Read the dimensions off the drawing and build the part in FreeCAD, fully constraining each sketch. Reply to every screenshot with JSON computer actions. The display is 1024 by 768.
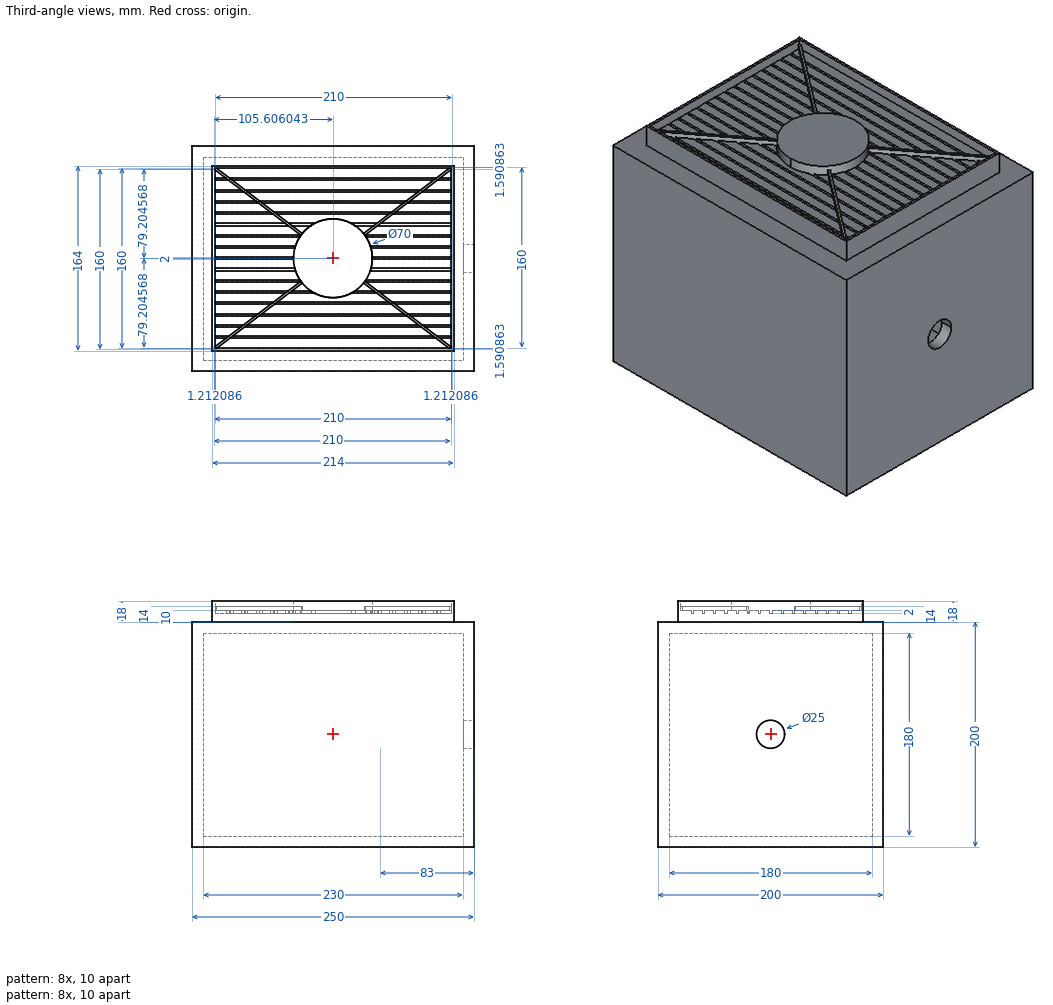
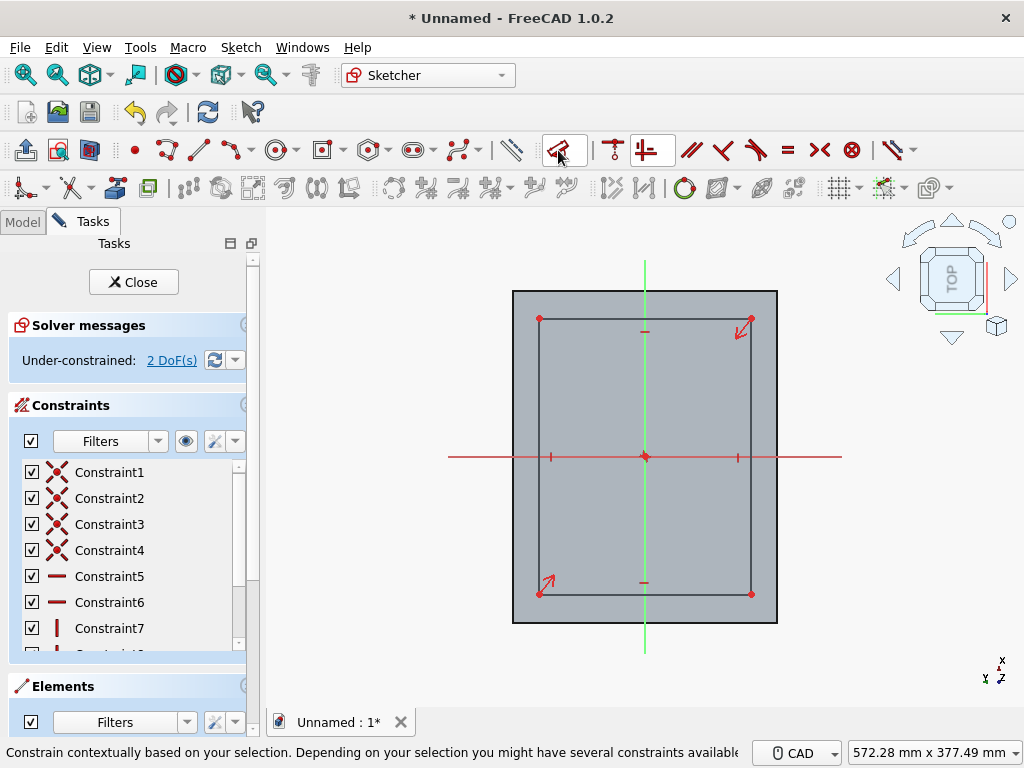
{"action": "left_click", "coordinate": [603, 595]}
{"action": "left_click", "coordinate": [596, 629]}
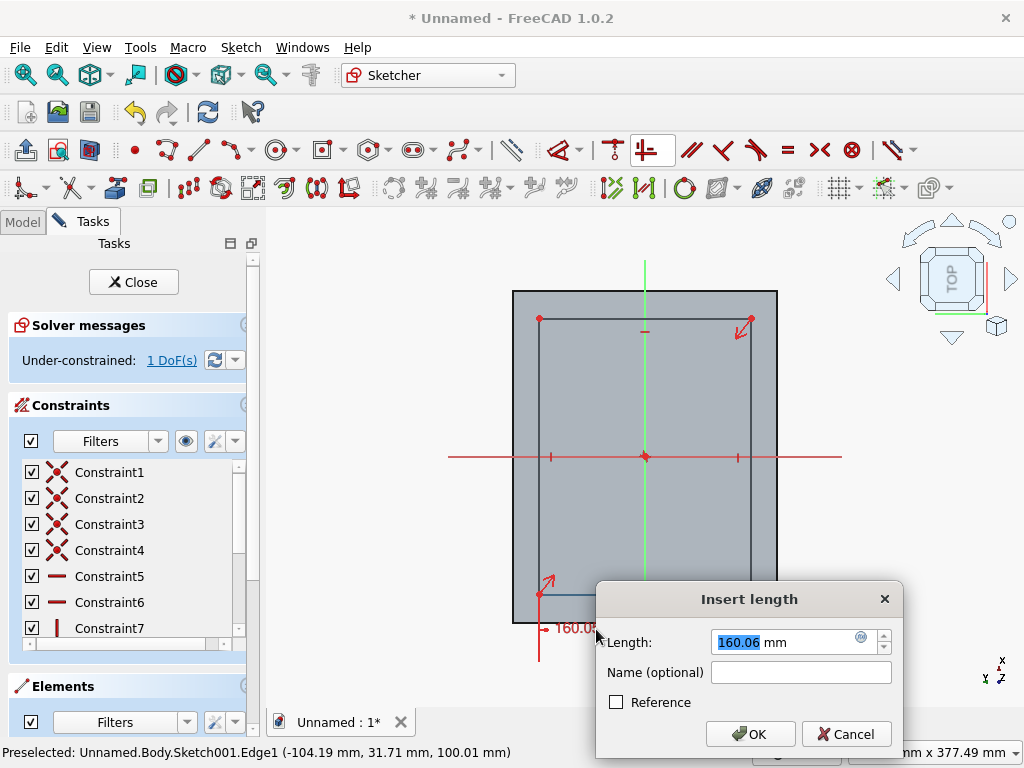
{"action": "type", "text": "160"}
{"action": "key", "text": "Return"}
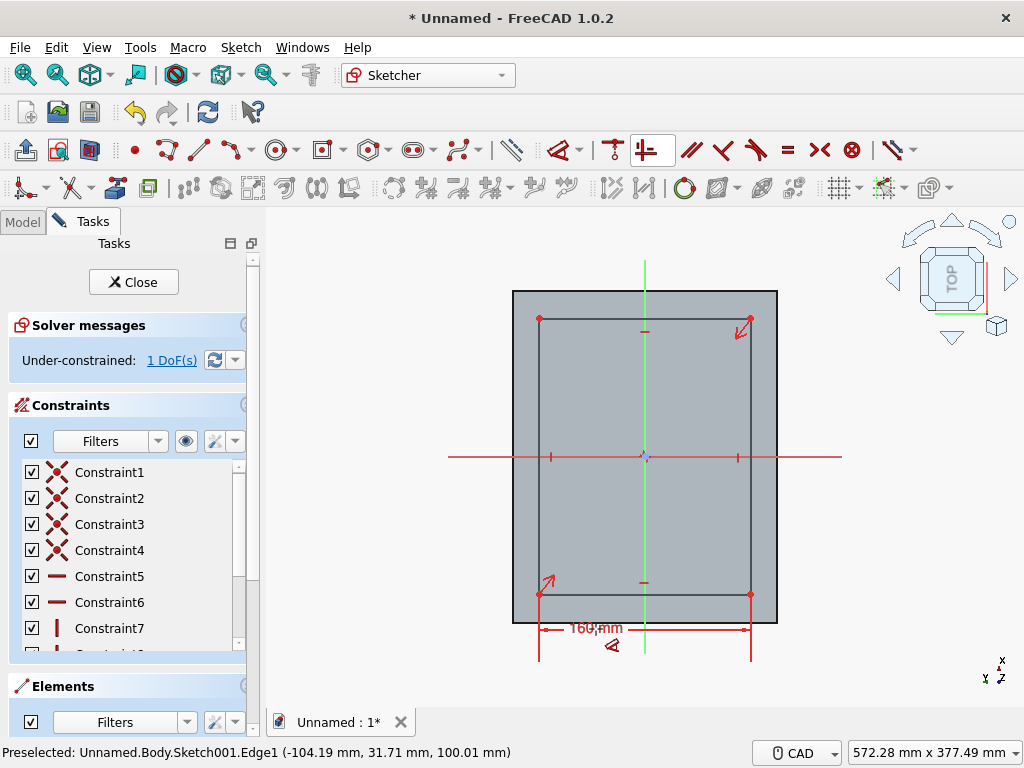
{"action": "left_click", "coordinate": [751, 512]}
{"action": "left_click", "coordinate": [785, 394]}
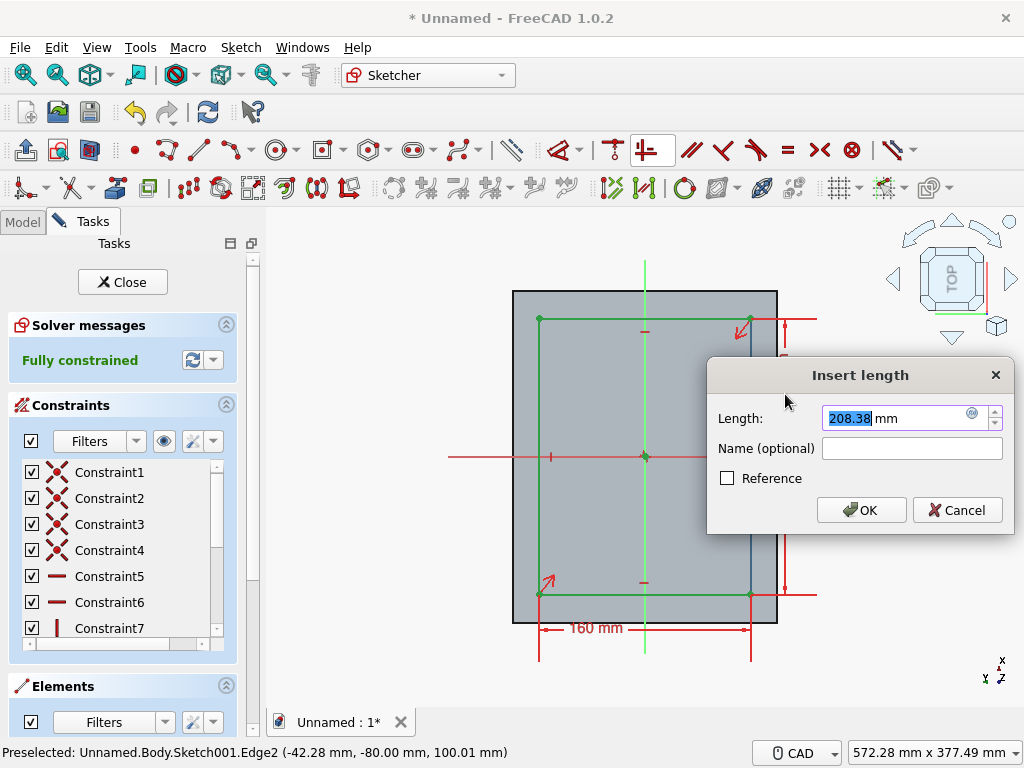
{"action": "type", "text": "210"}
{"action": "key", "text": "Return"}
{"action": "key", "text": "Escape"}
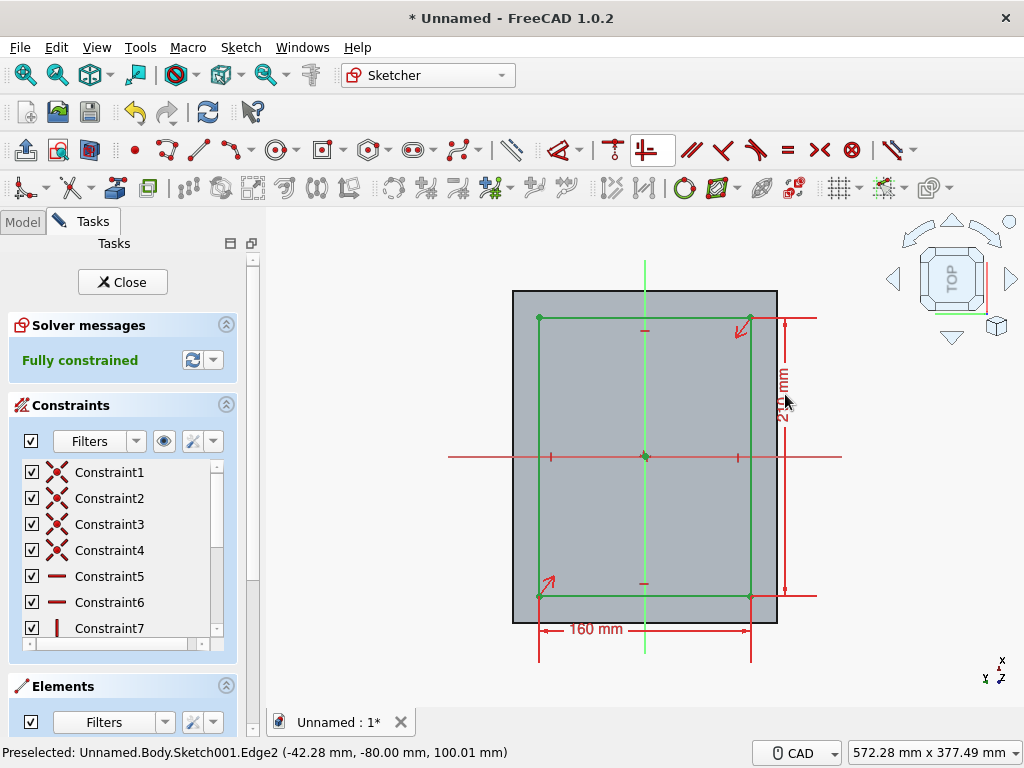
{"action": "left_click", "coordinate": [123, 282]}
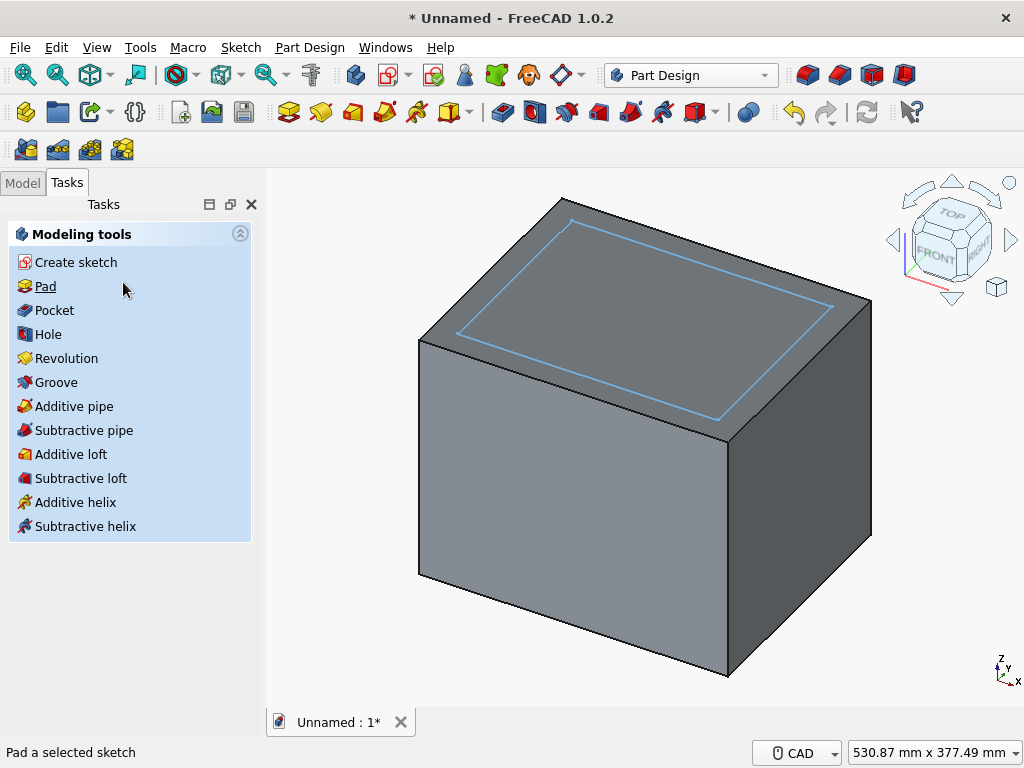
{"action": "left_click", "coordinate": [290, 112]}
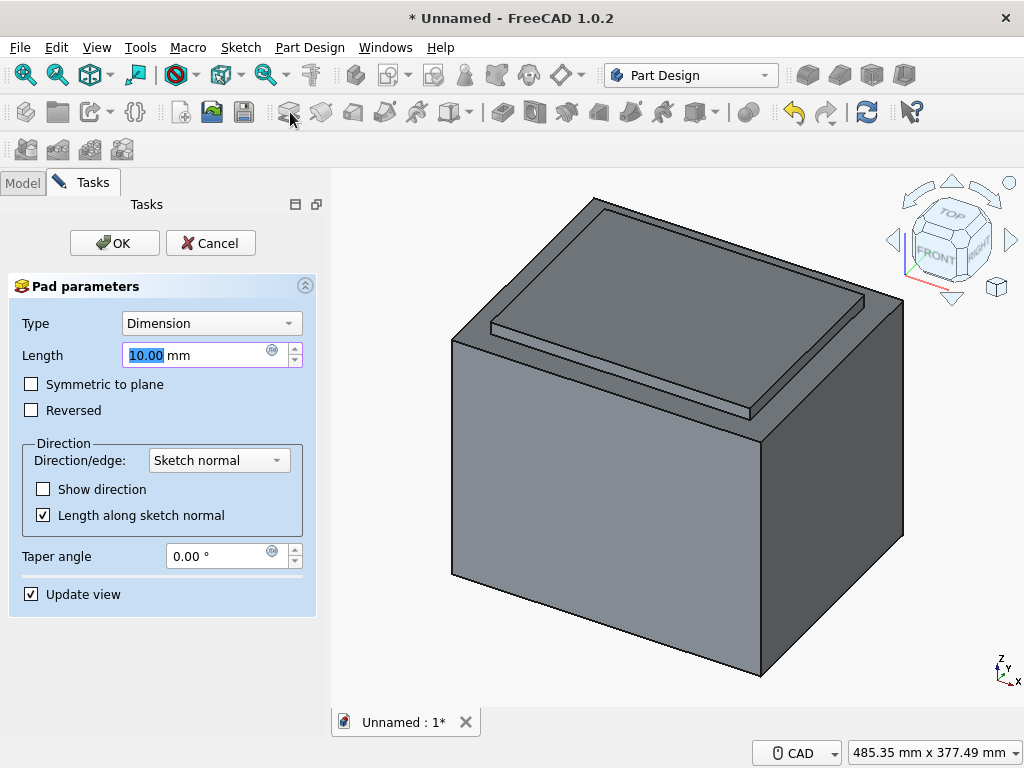
{"action": "type", "text": "10"}
{"action": "key", "text": "Tab"}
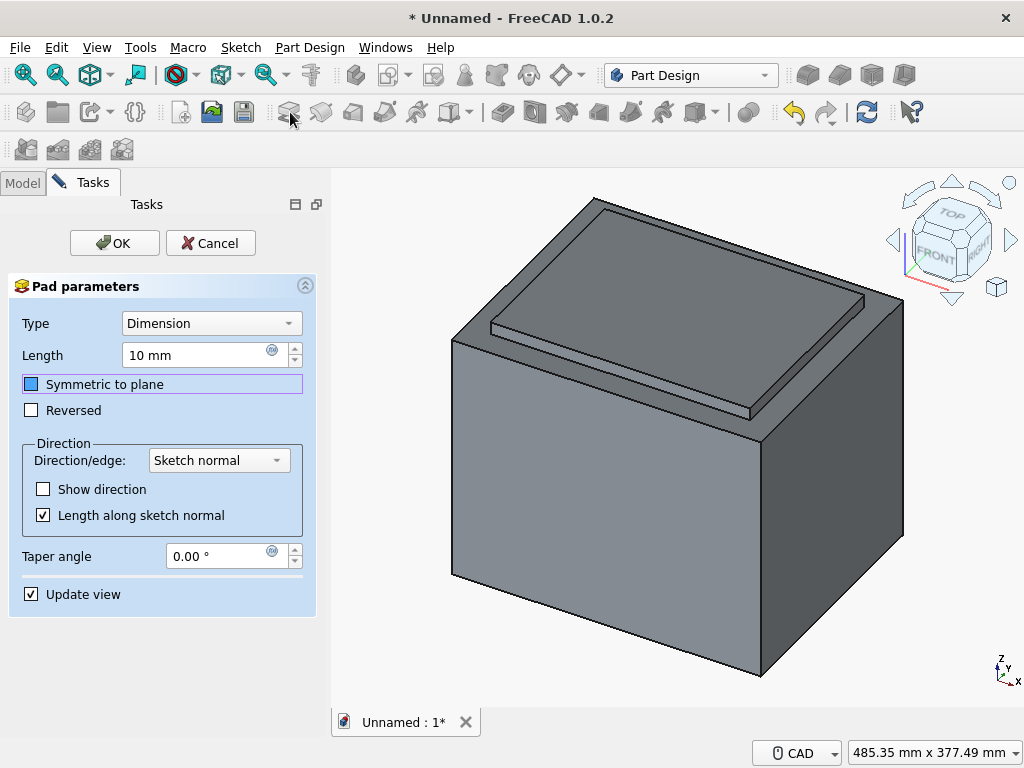
{"action": "left_click", "coordinate": [115, 243]}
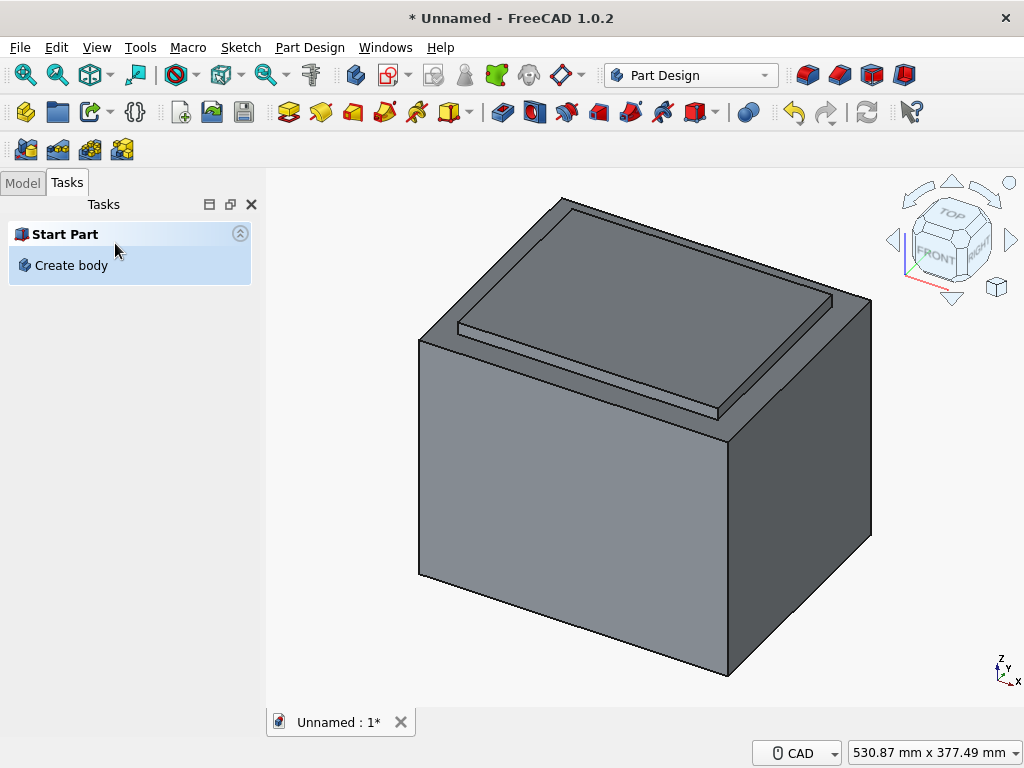
{"action": "left_click", "coordinate": [645, 308]}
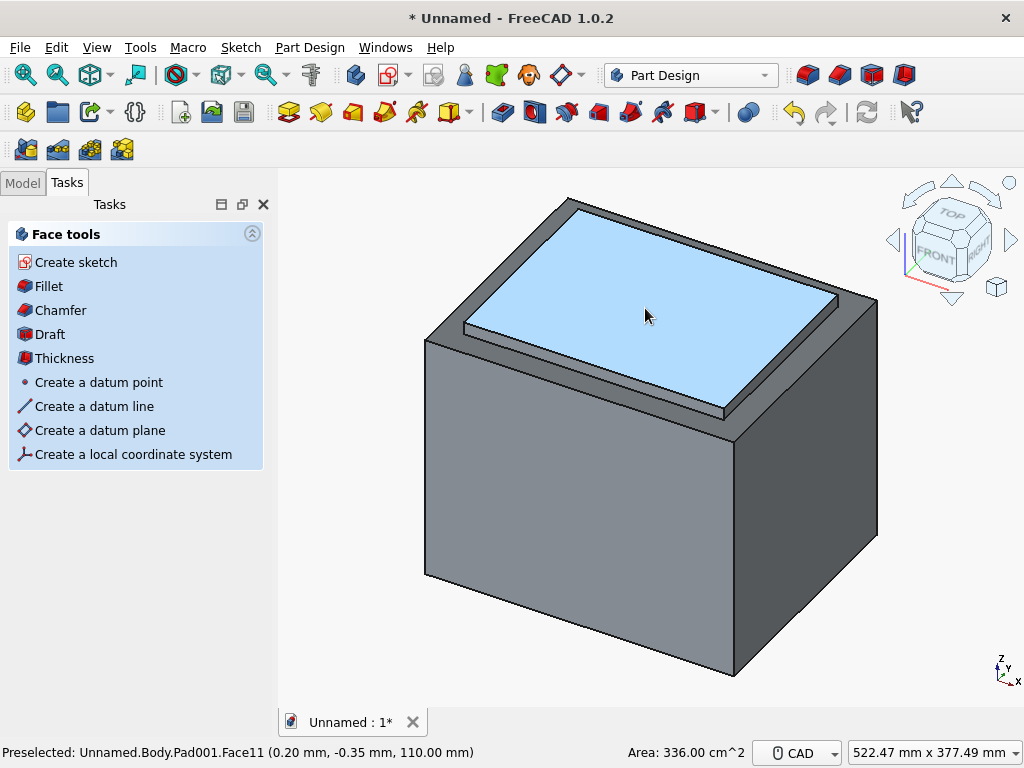
{"action": "left_click", "coordinate": [388, 76]}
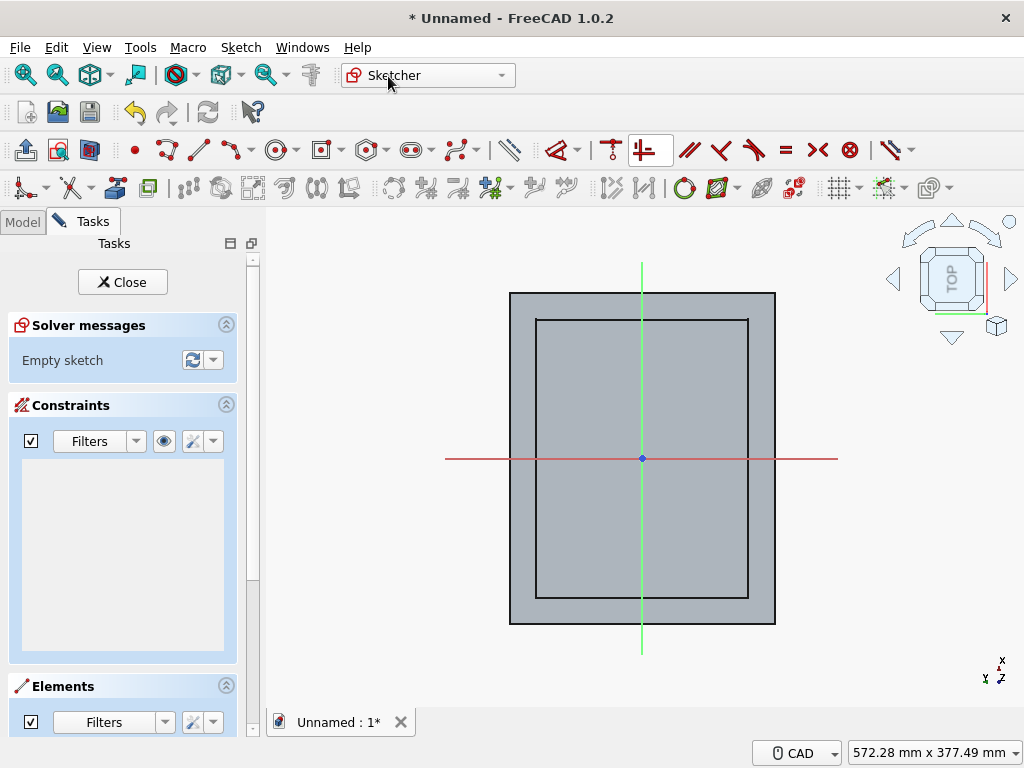
{"action": "left_click", "coordinate": [322, 150]}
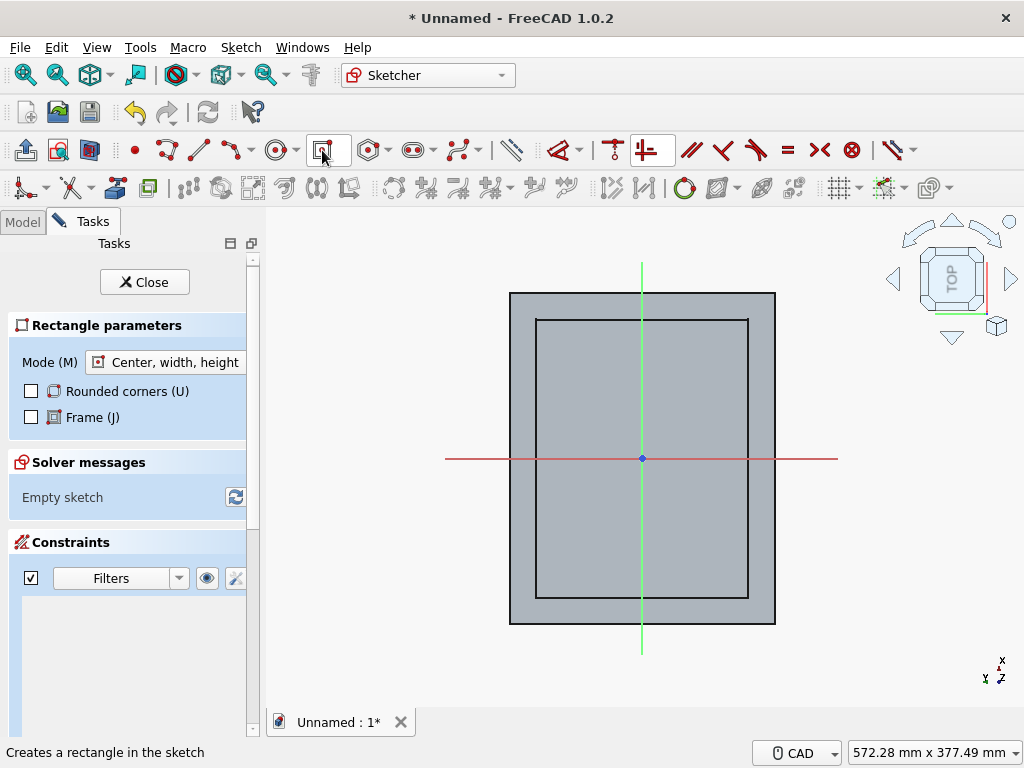
{"action": "scroll", "coordinate": [642, 459], "scroll_direction": "up", "scroll_amount": 13}